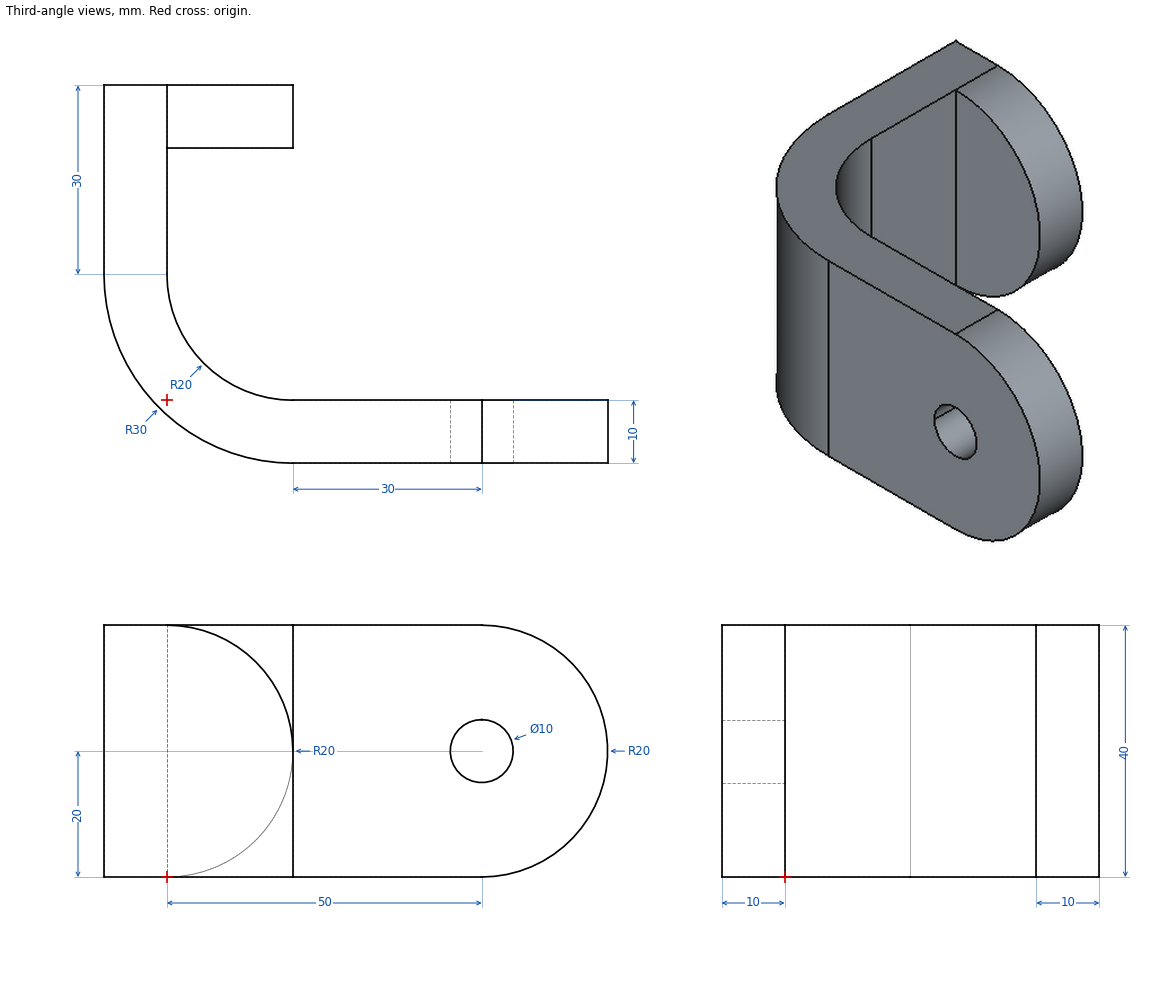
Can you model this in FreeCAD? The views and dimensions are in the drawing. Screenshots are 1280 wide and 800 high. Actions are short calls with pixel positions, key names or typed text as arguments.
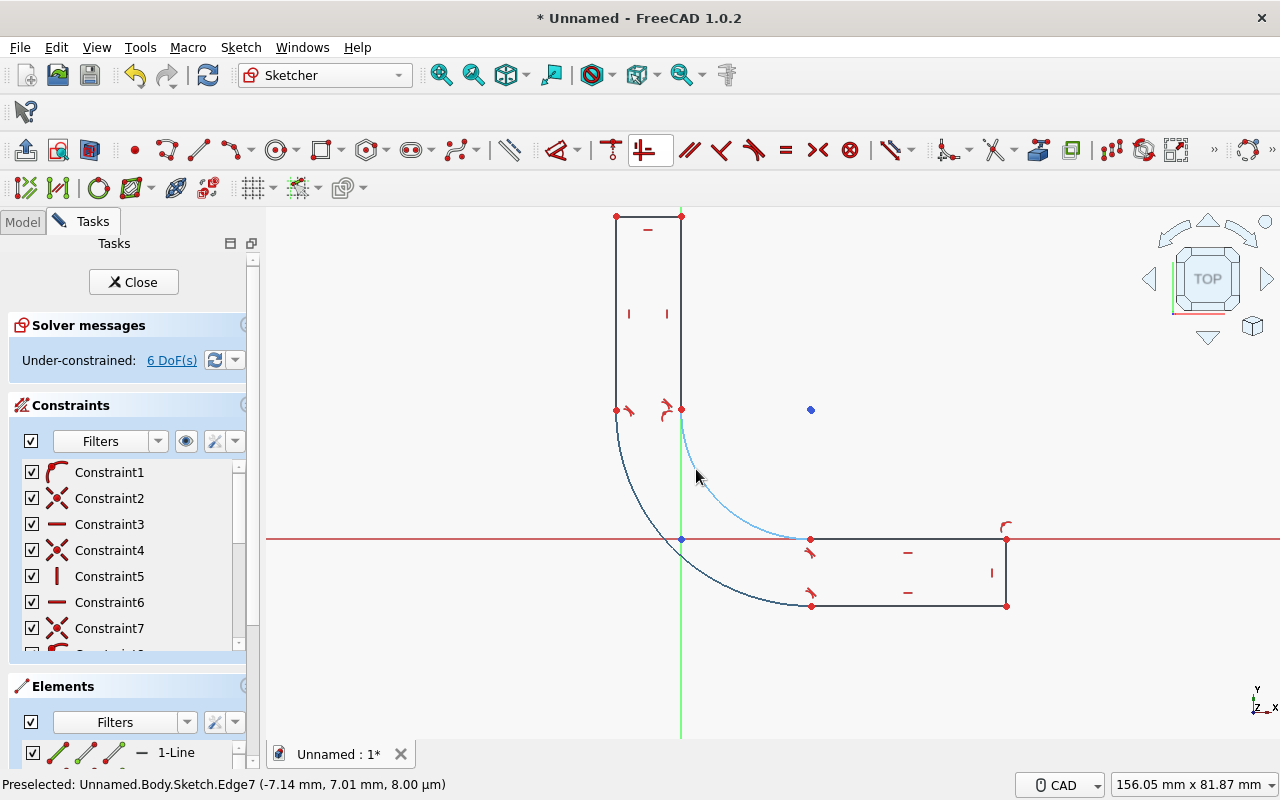
click(695, 469)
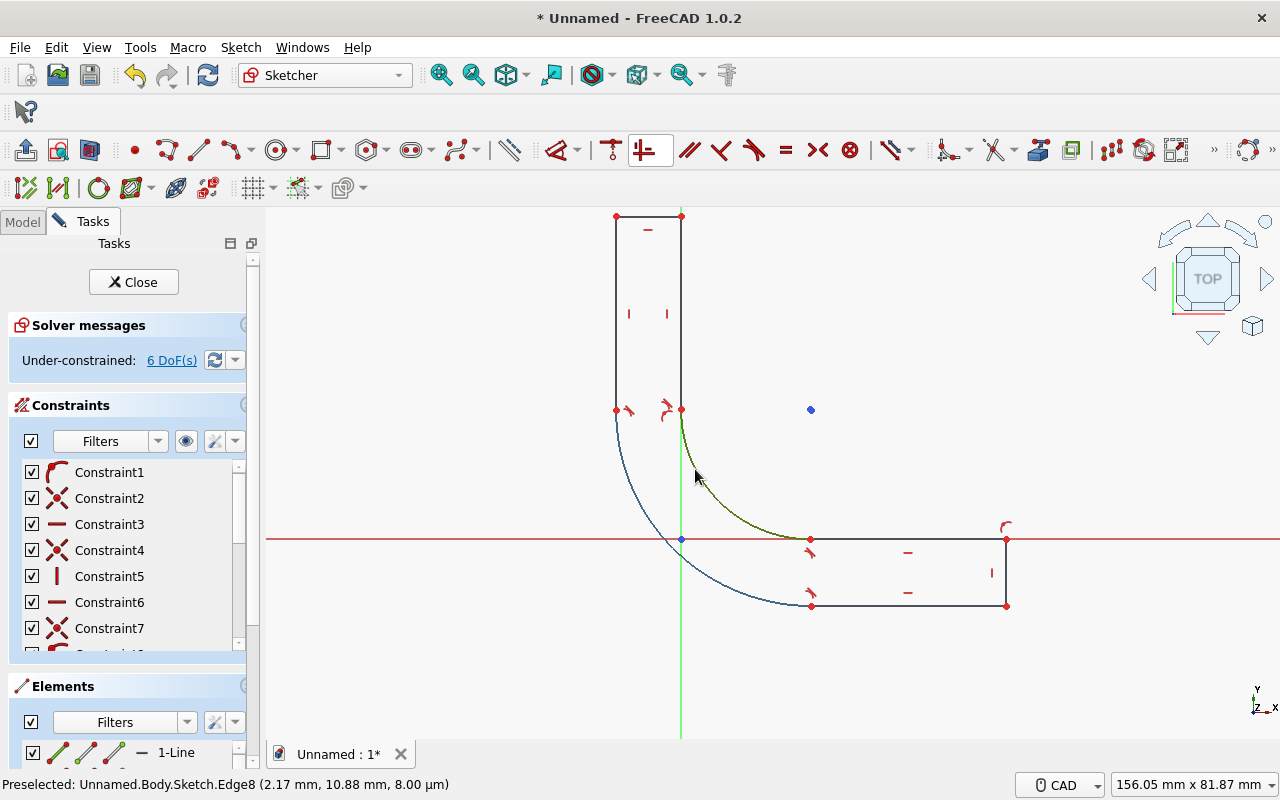
click(612, 150)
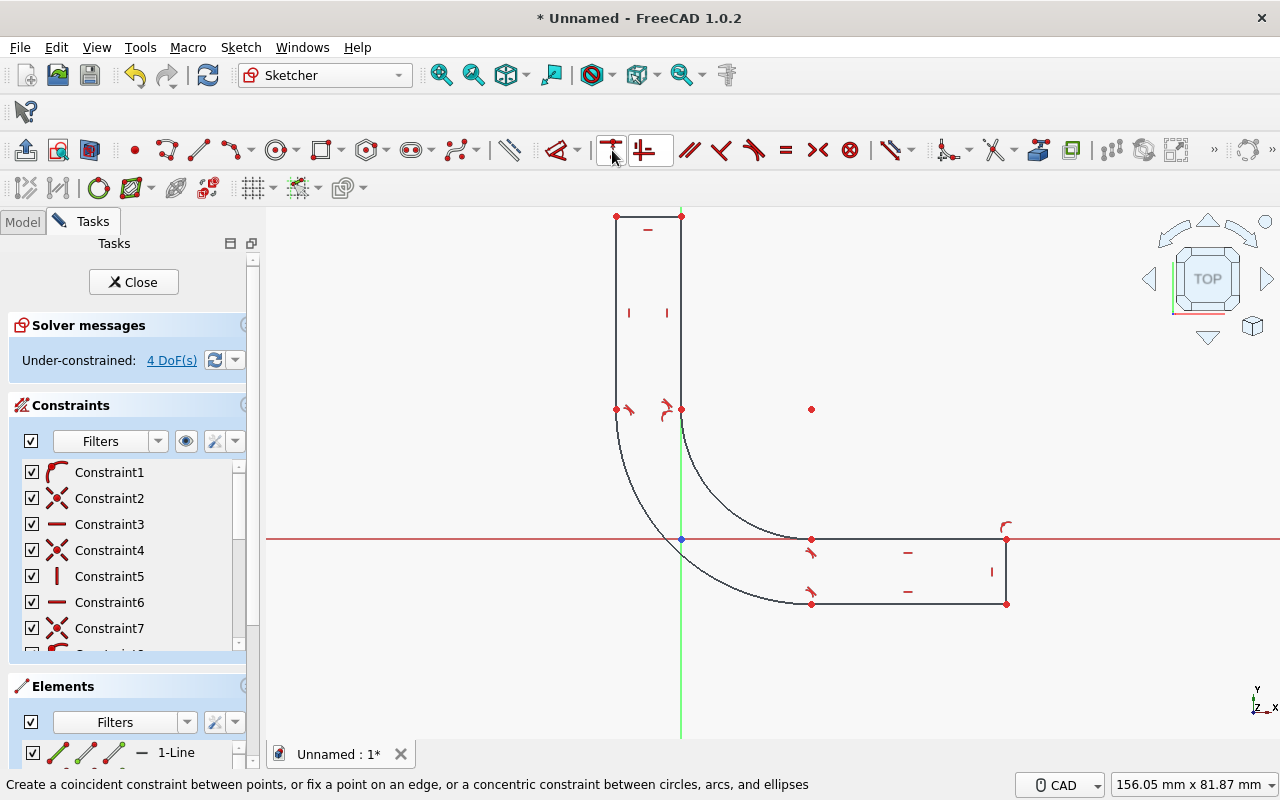
key(d)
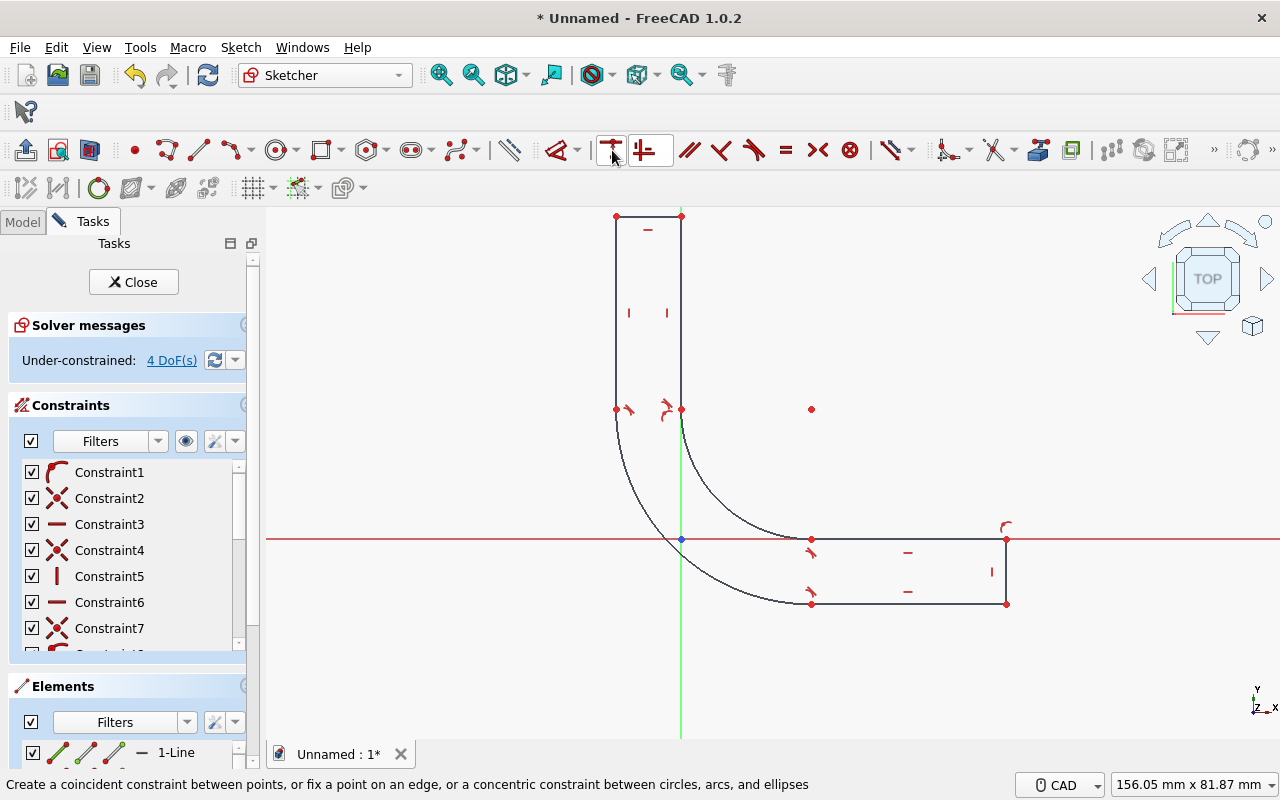
click(637, 498)
click(608, 513)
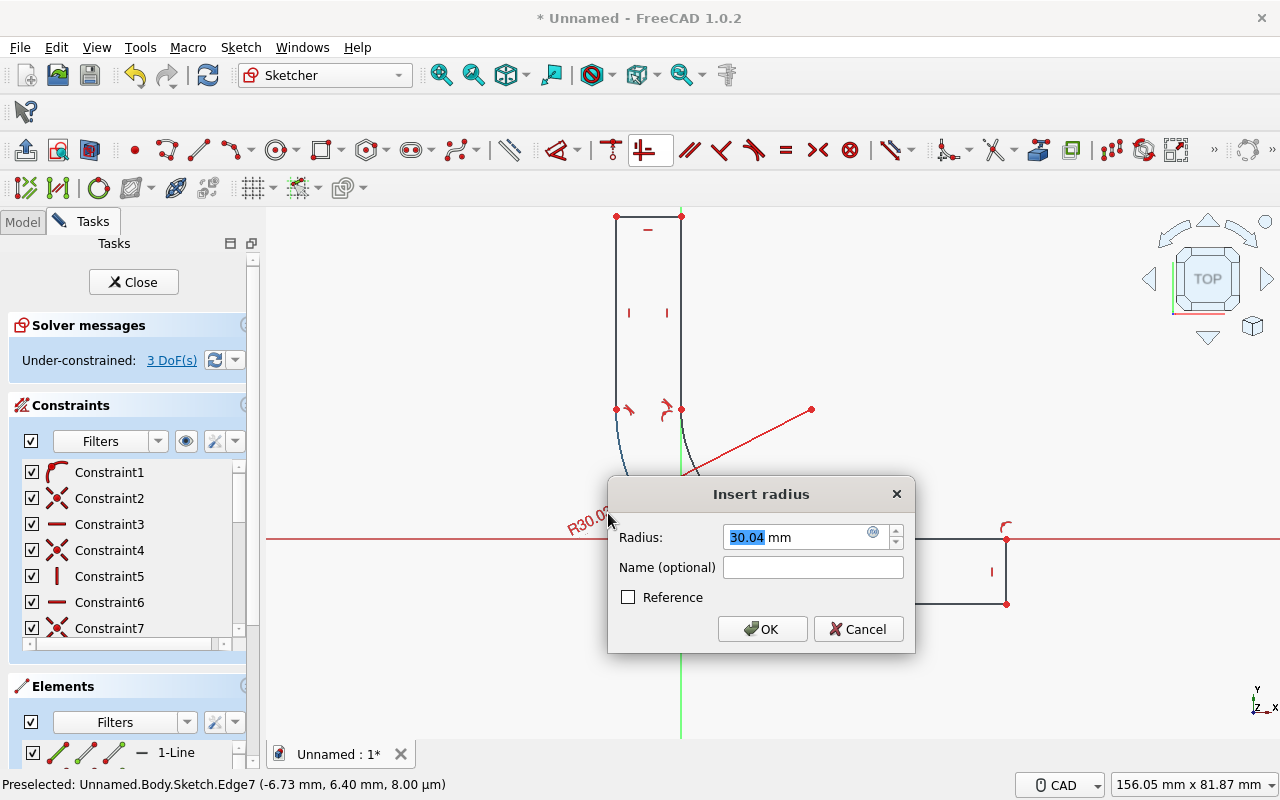
text(30)
key(Return)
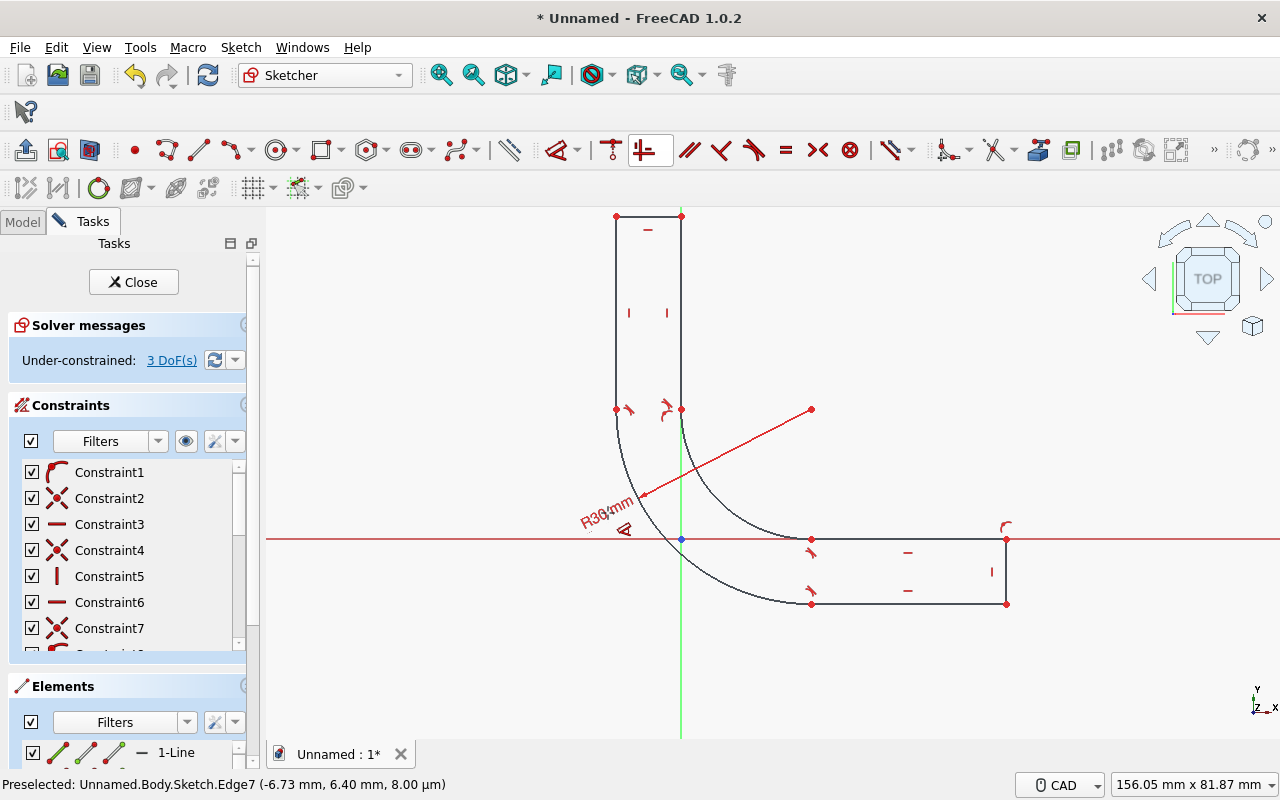
click(695, 468)
click(666, 482)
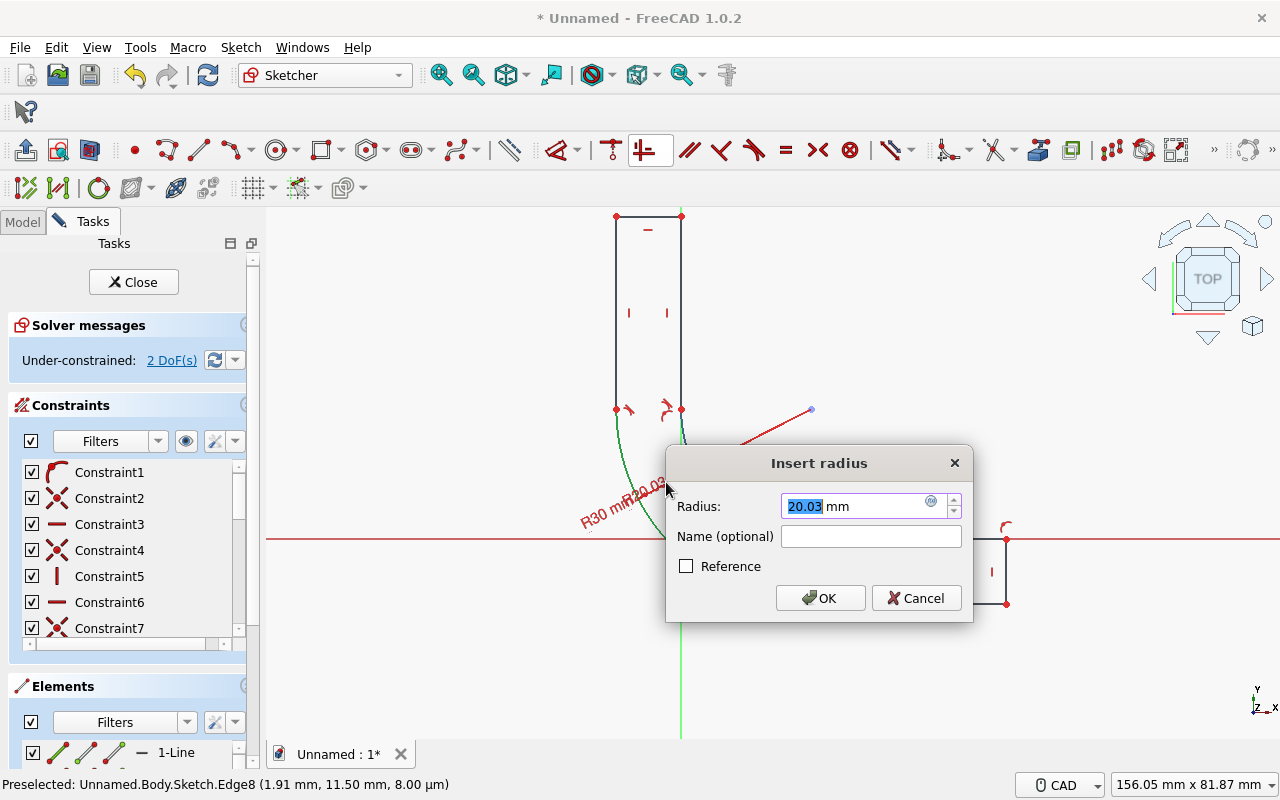
text(20)
key(Return)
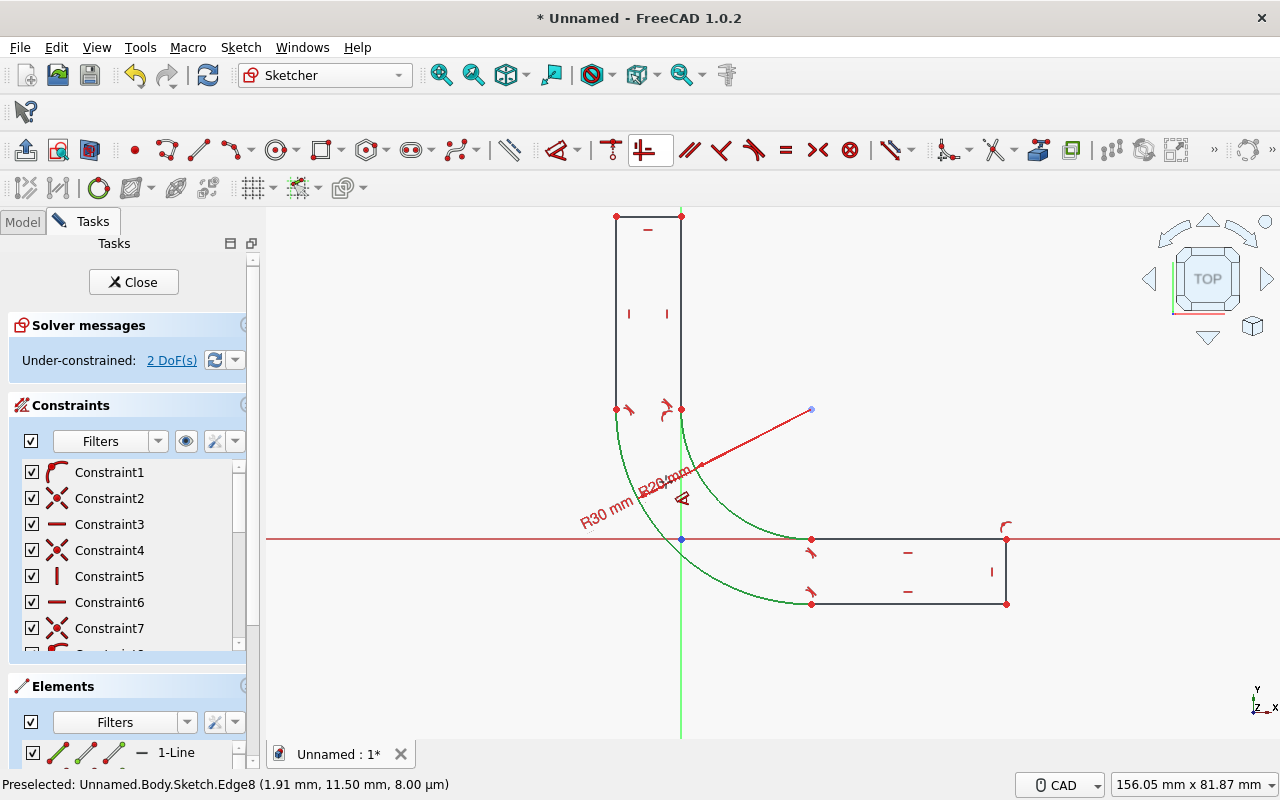
click(681, 352)
click(647, 322)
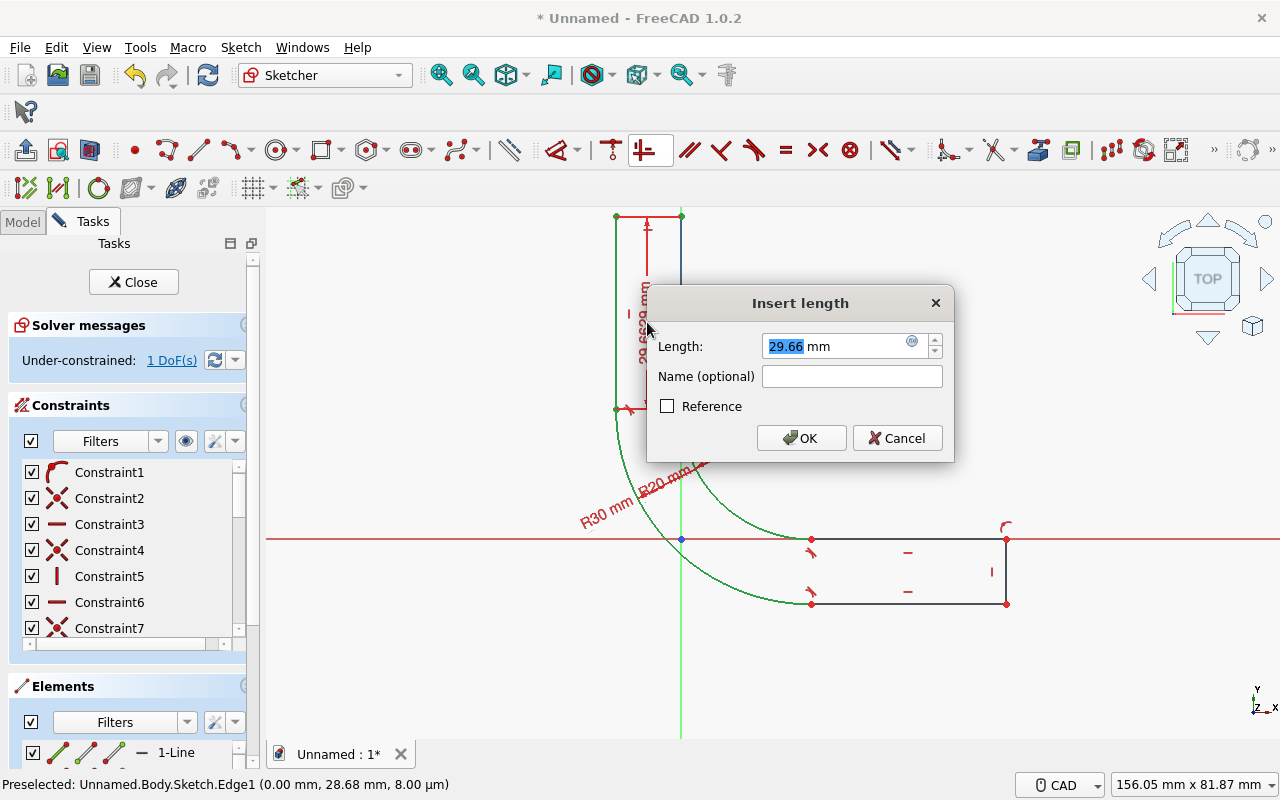
text(30)
key(Return)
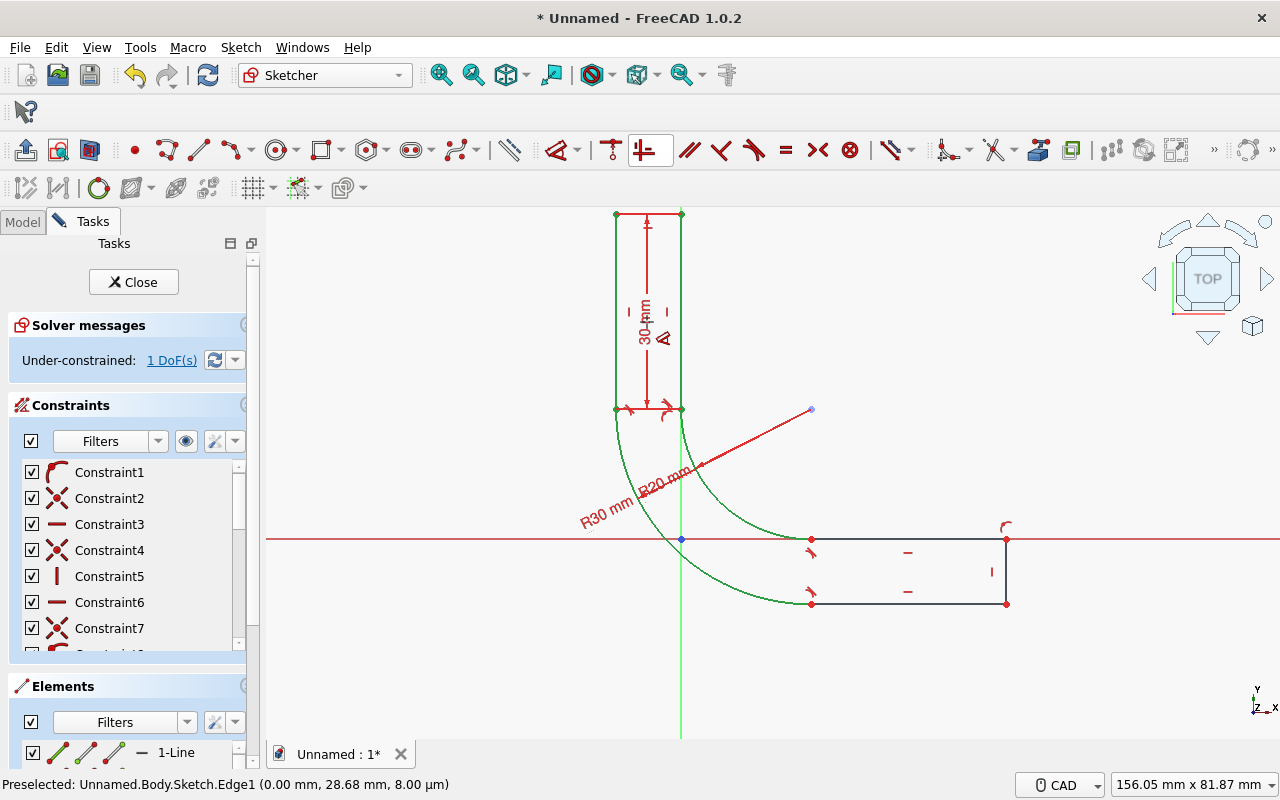
click(870, 604)
click(909, 638)